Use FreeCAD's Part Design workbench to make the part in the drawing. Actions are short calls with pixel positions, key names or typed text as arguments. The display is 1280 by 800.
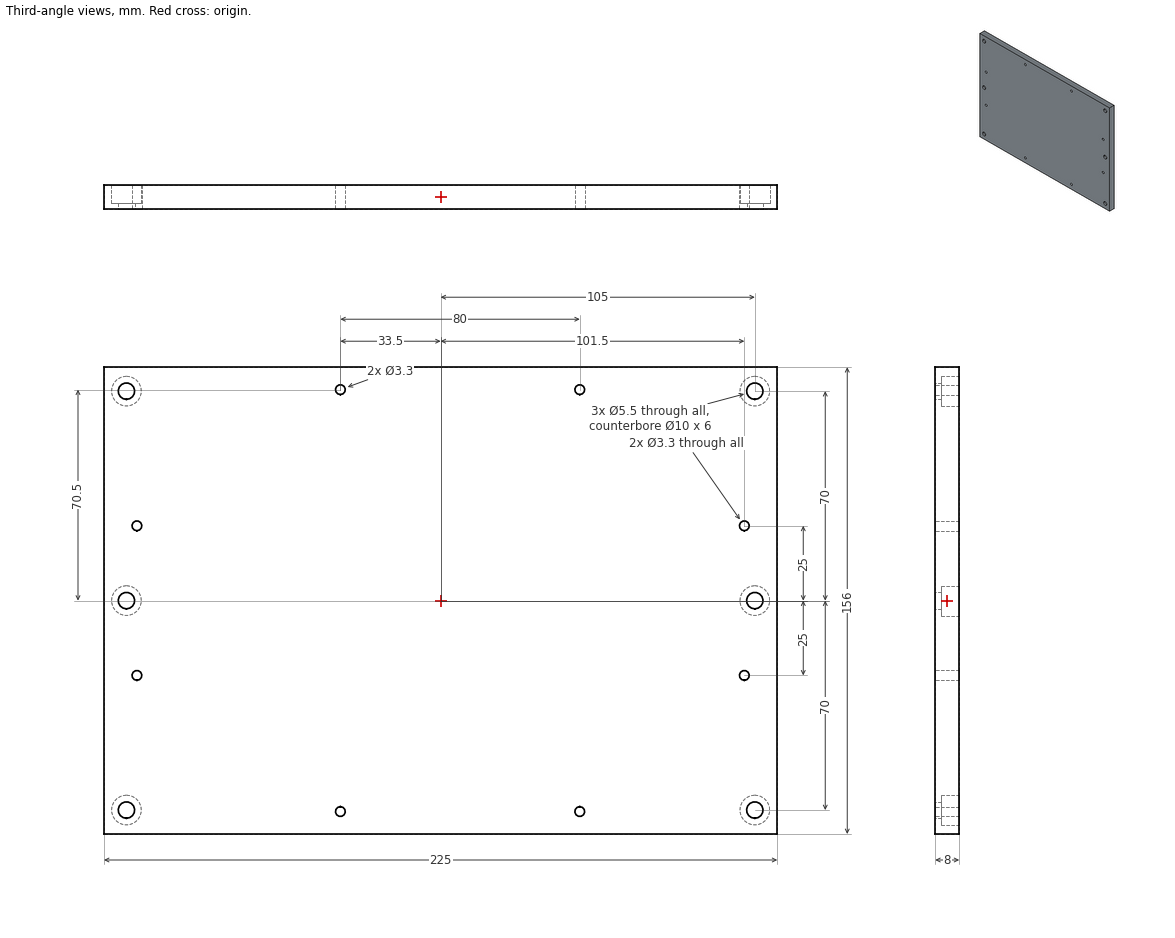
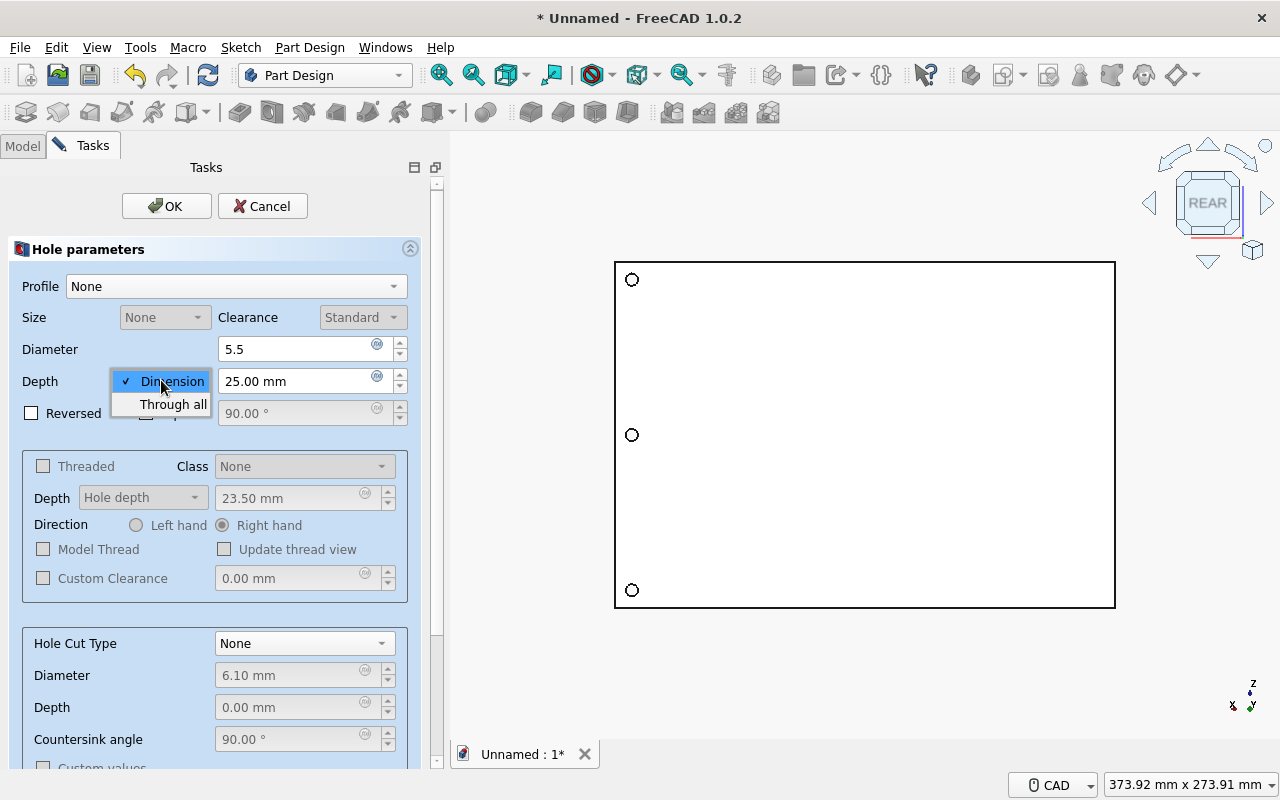
click(160, 404)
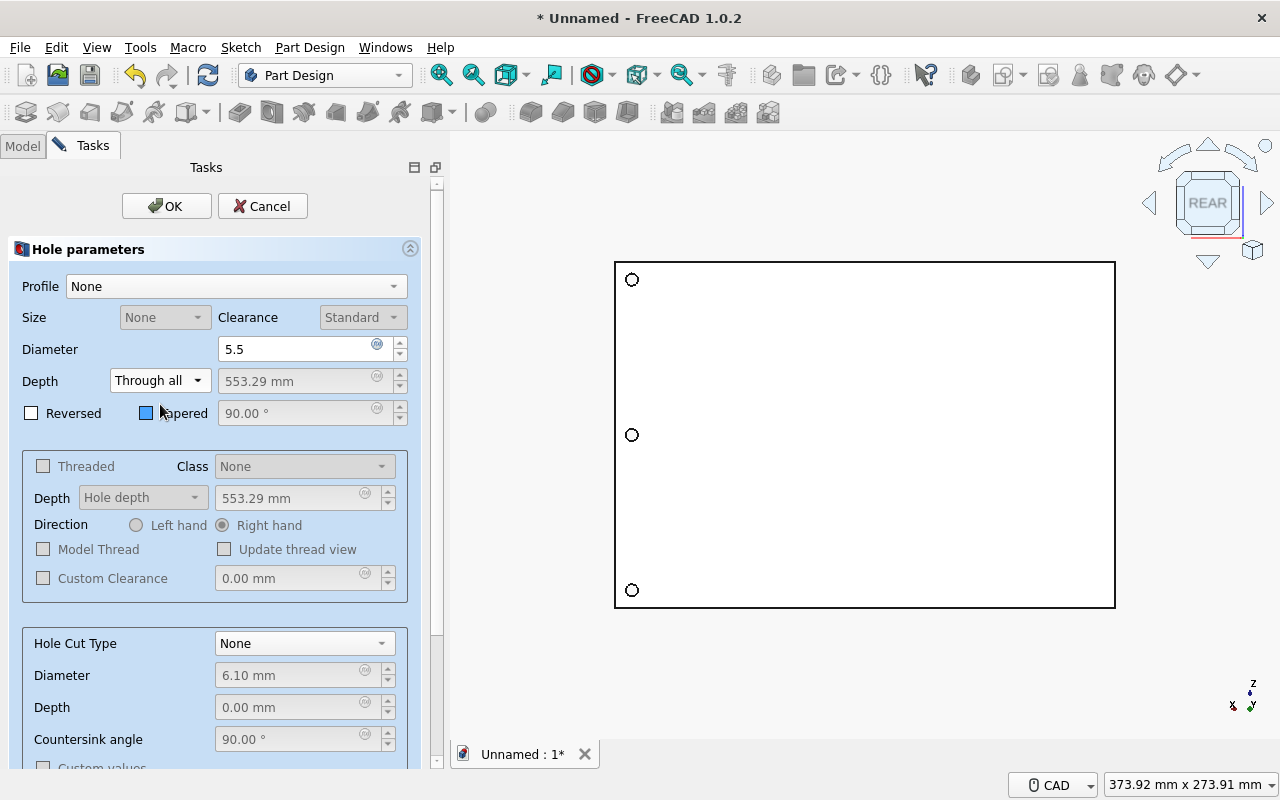
click(306, 644)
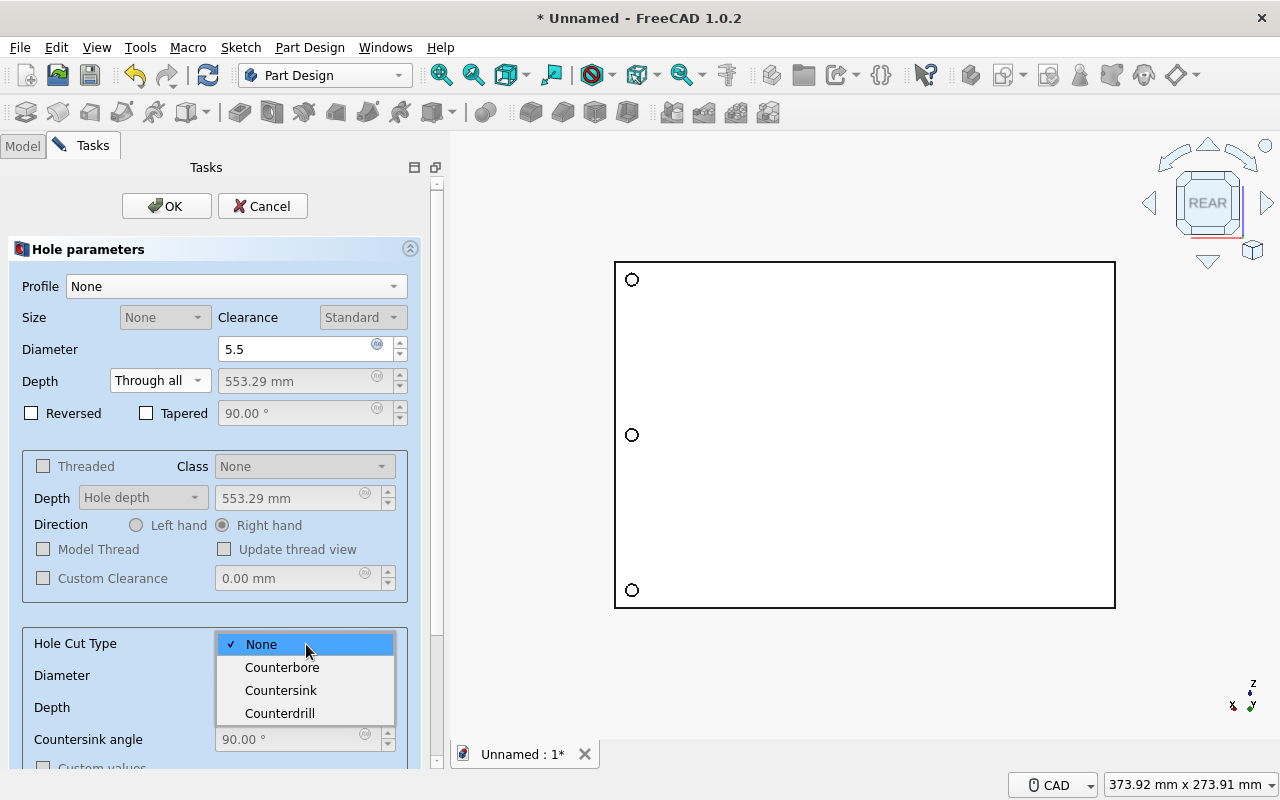
click(304, 668)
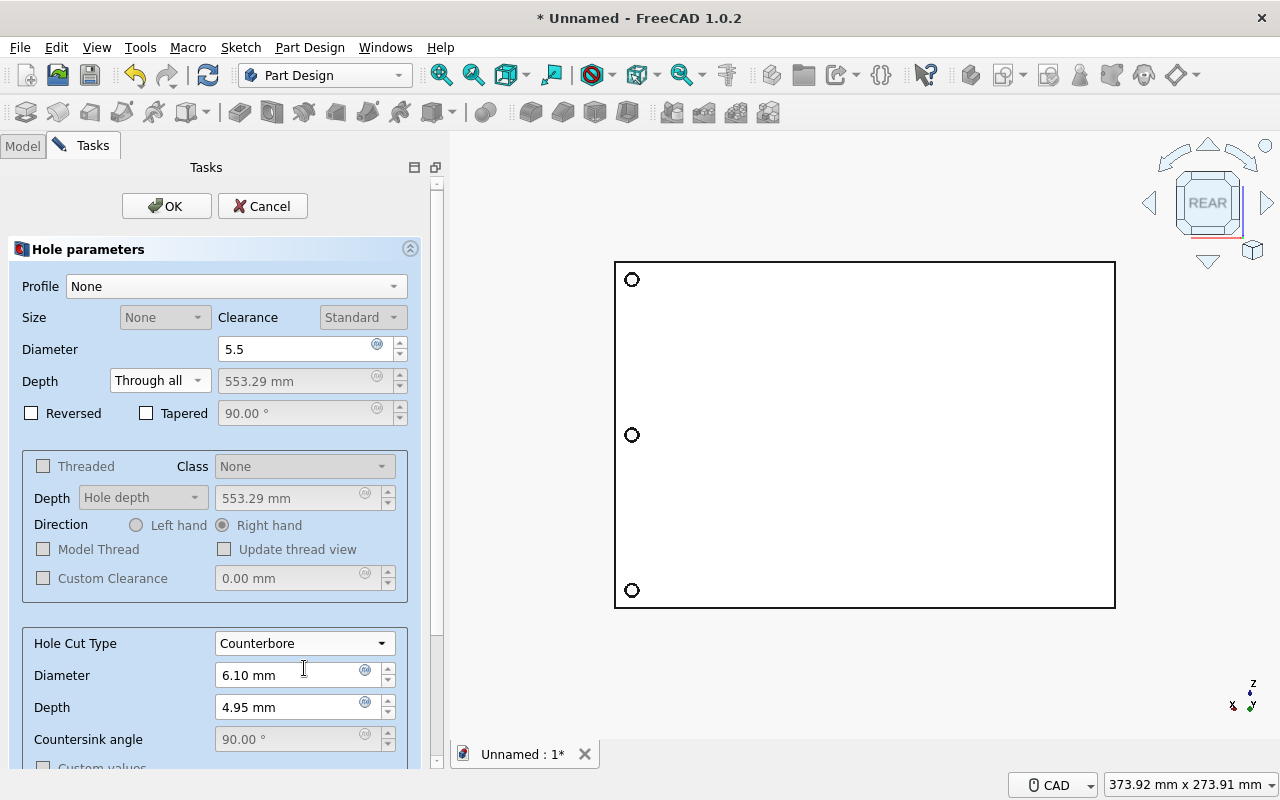
triple_click(298, 675)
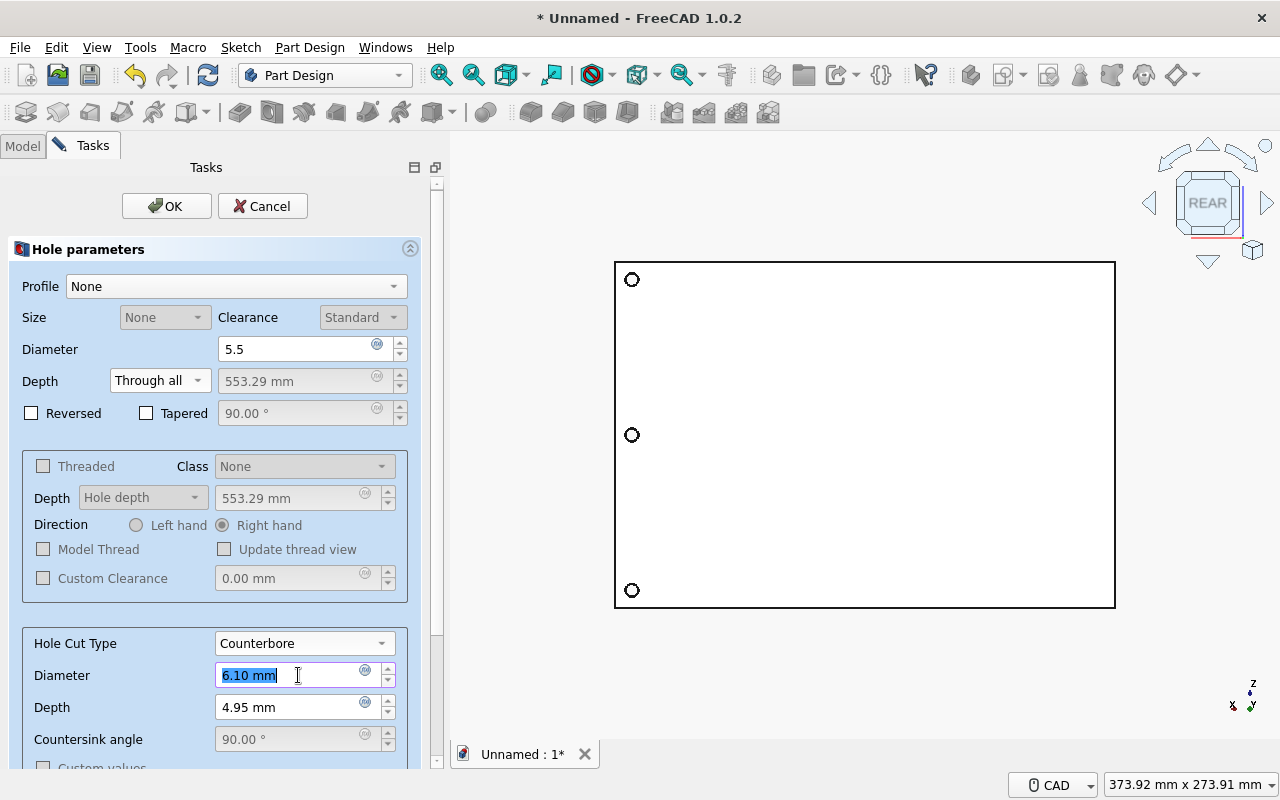
text(10)
key(Tab)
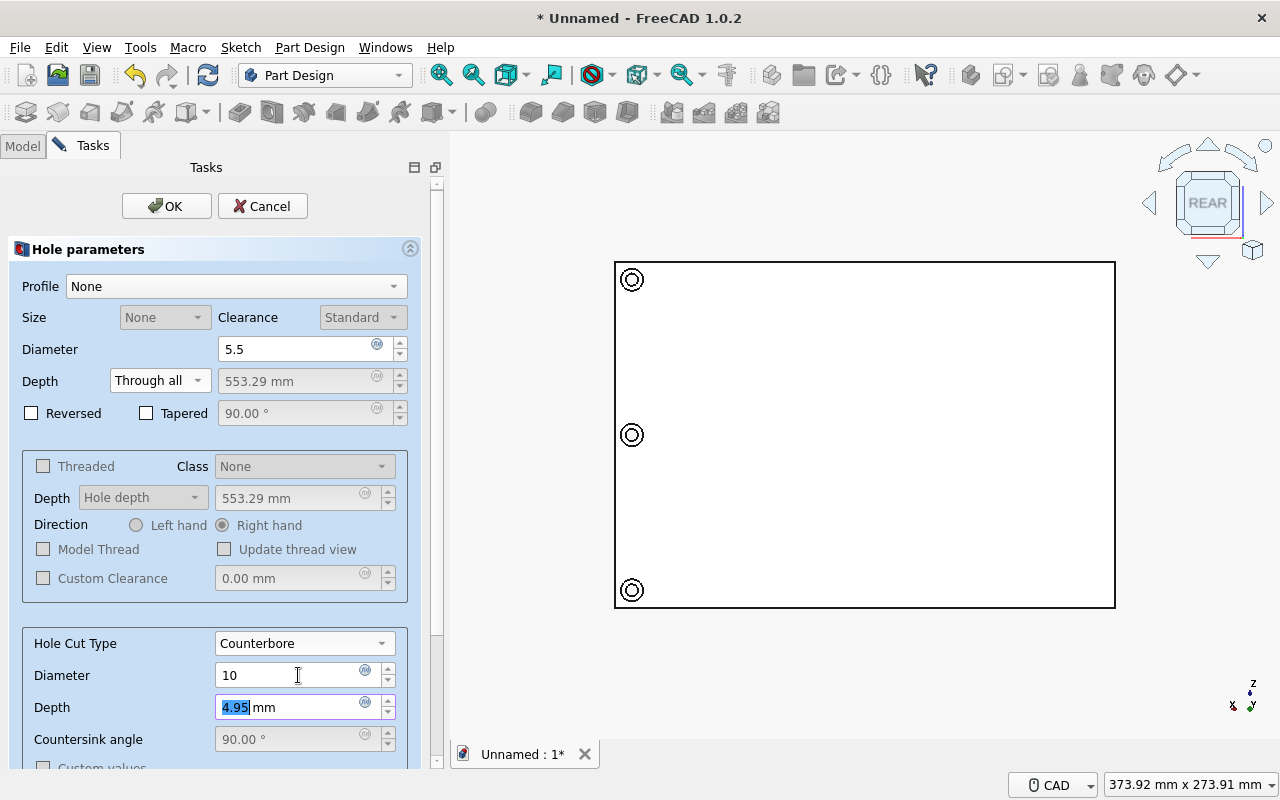
text(6)
key(Tab)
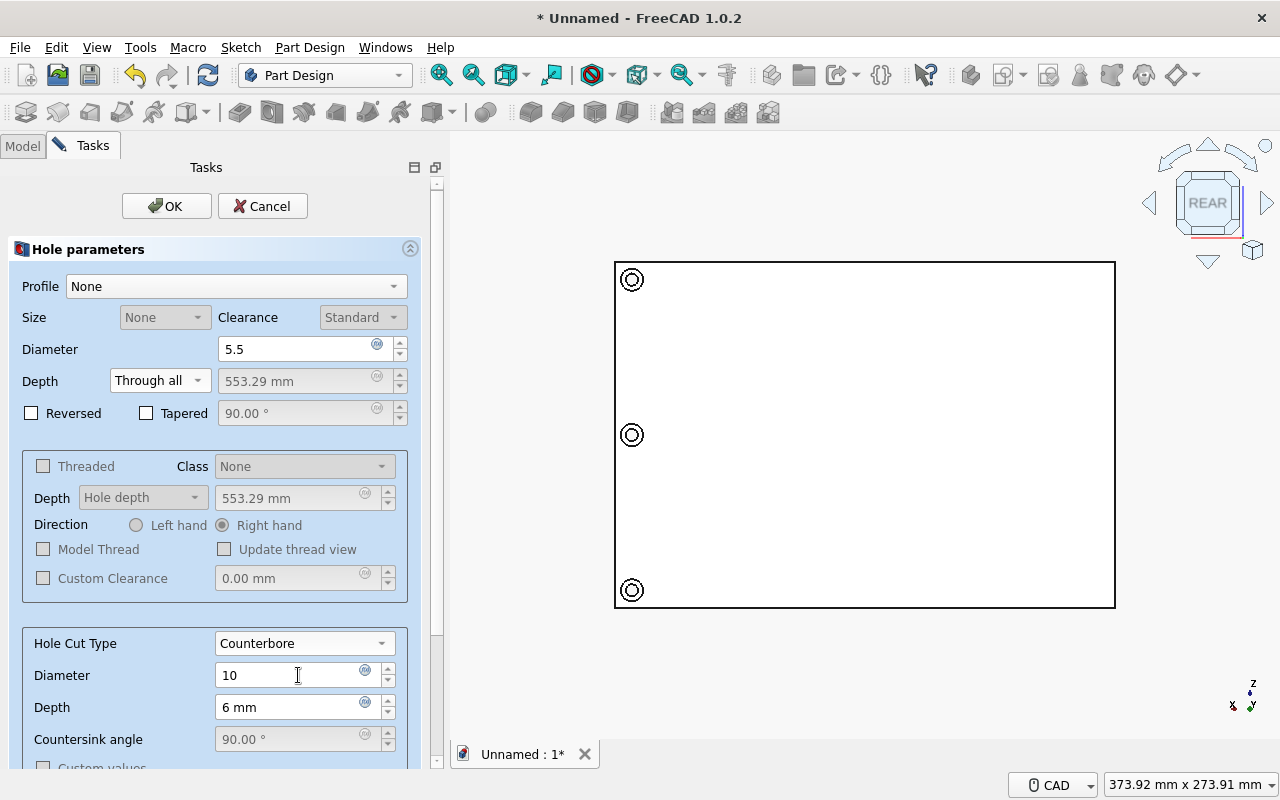
click(167, 206)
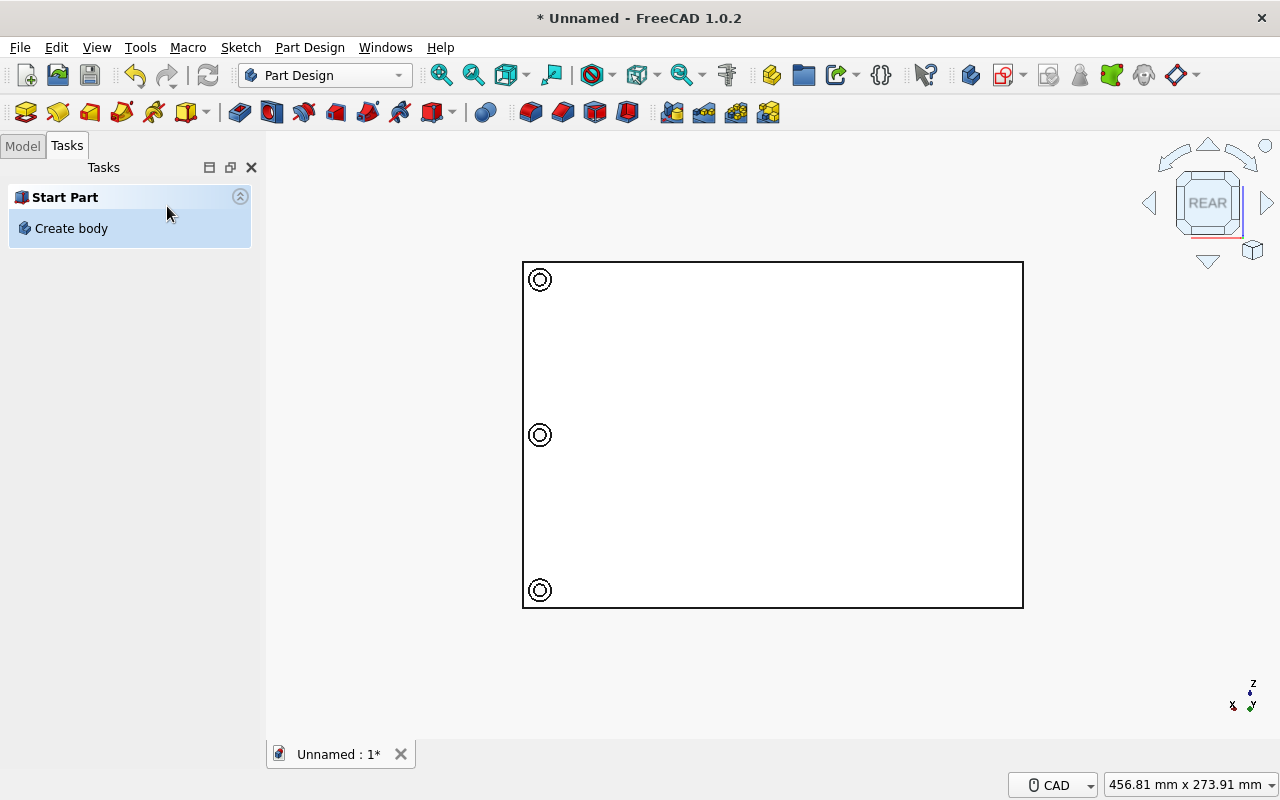
click(23, 145)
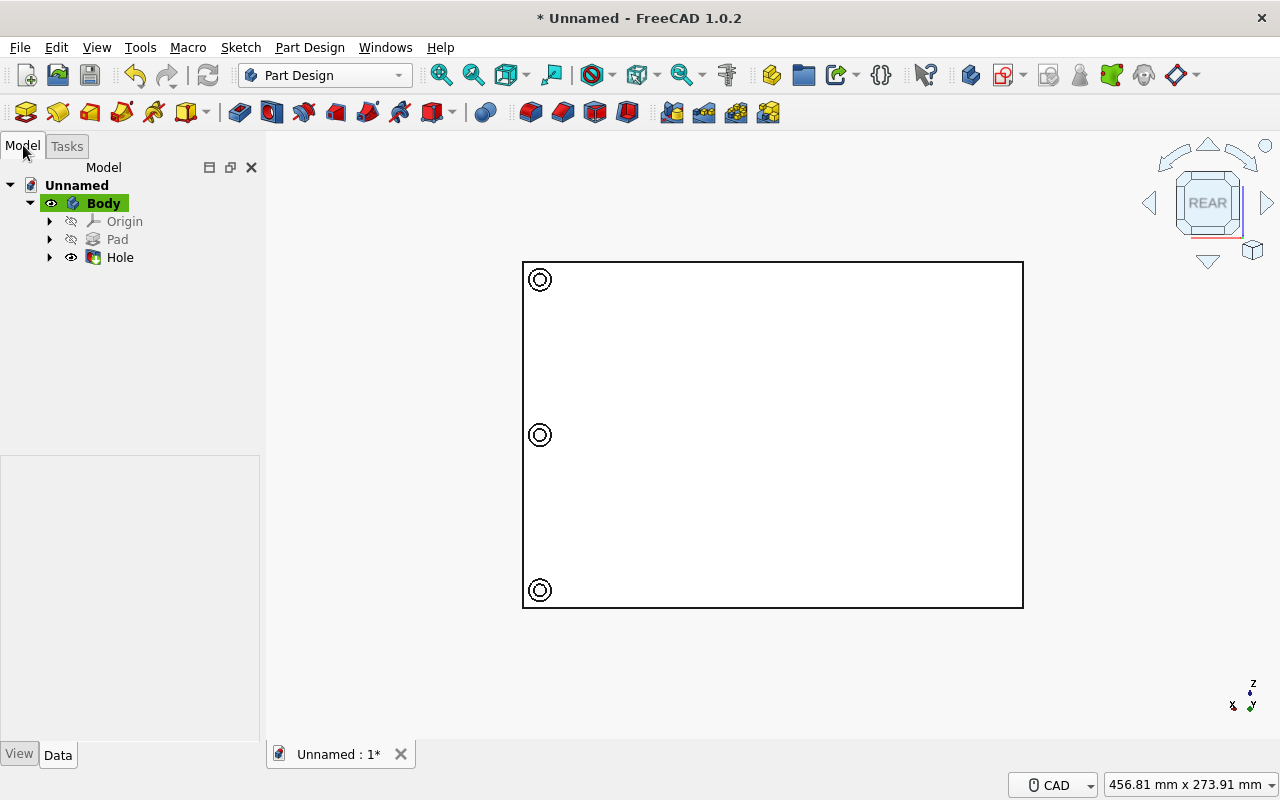
click(116, 257)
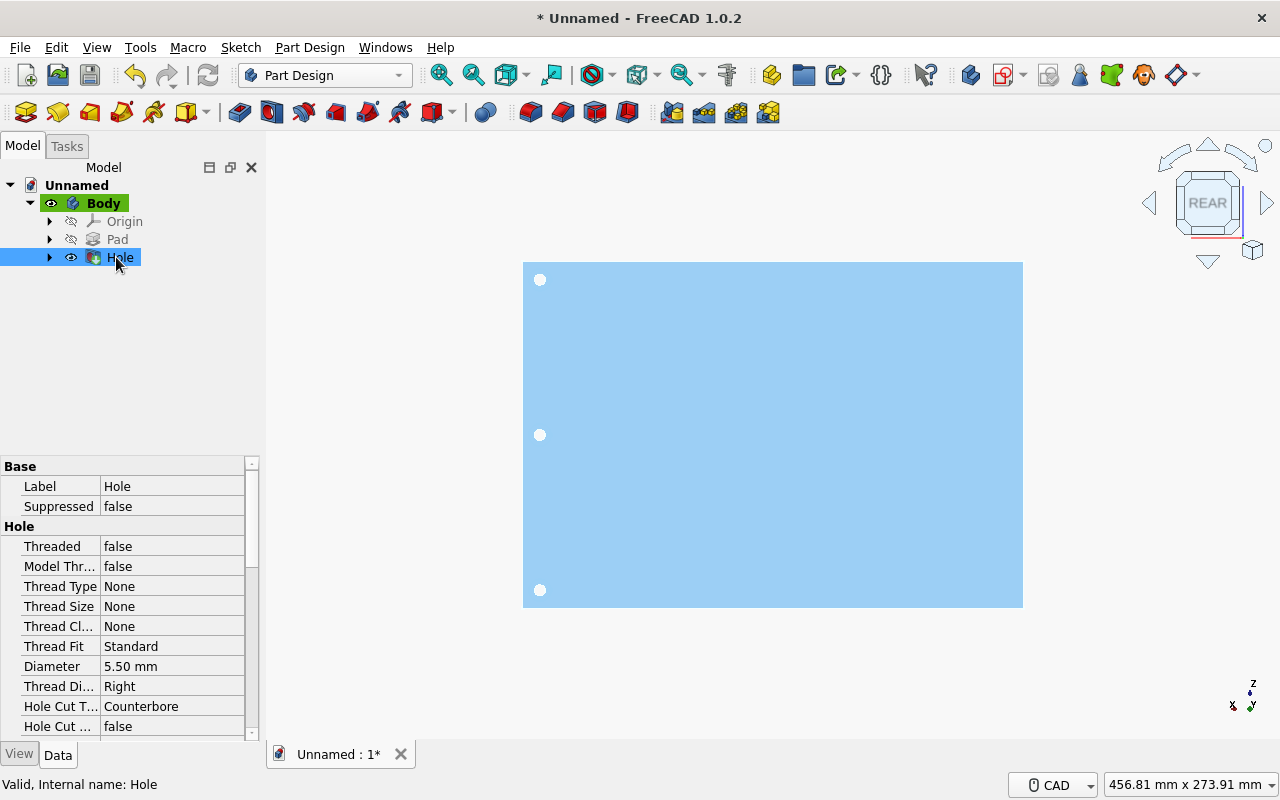
click(672, 112)